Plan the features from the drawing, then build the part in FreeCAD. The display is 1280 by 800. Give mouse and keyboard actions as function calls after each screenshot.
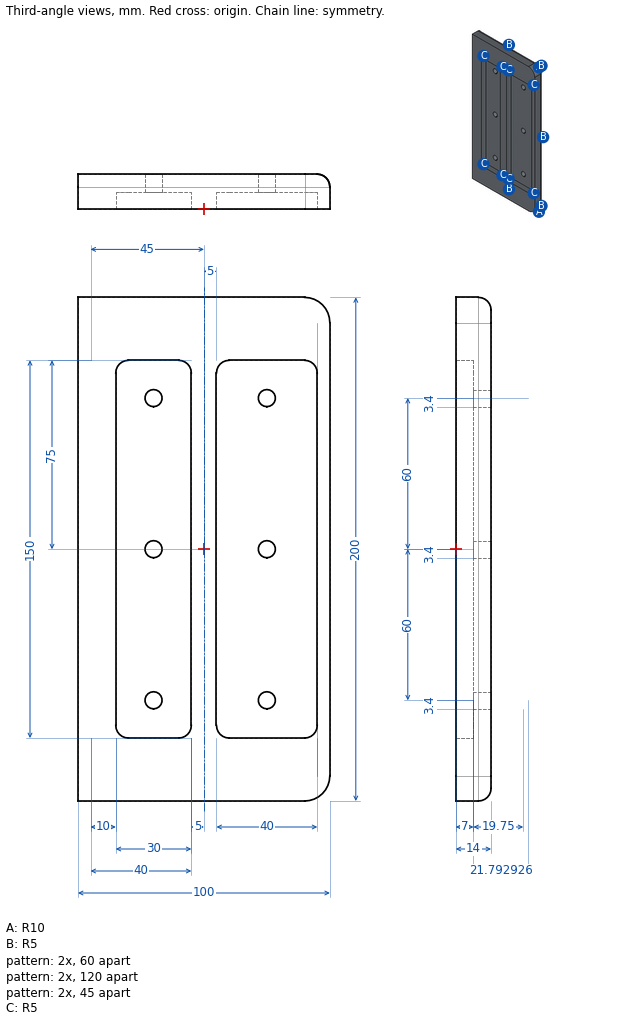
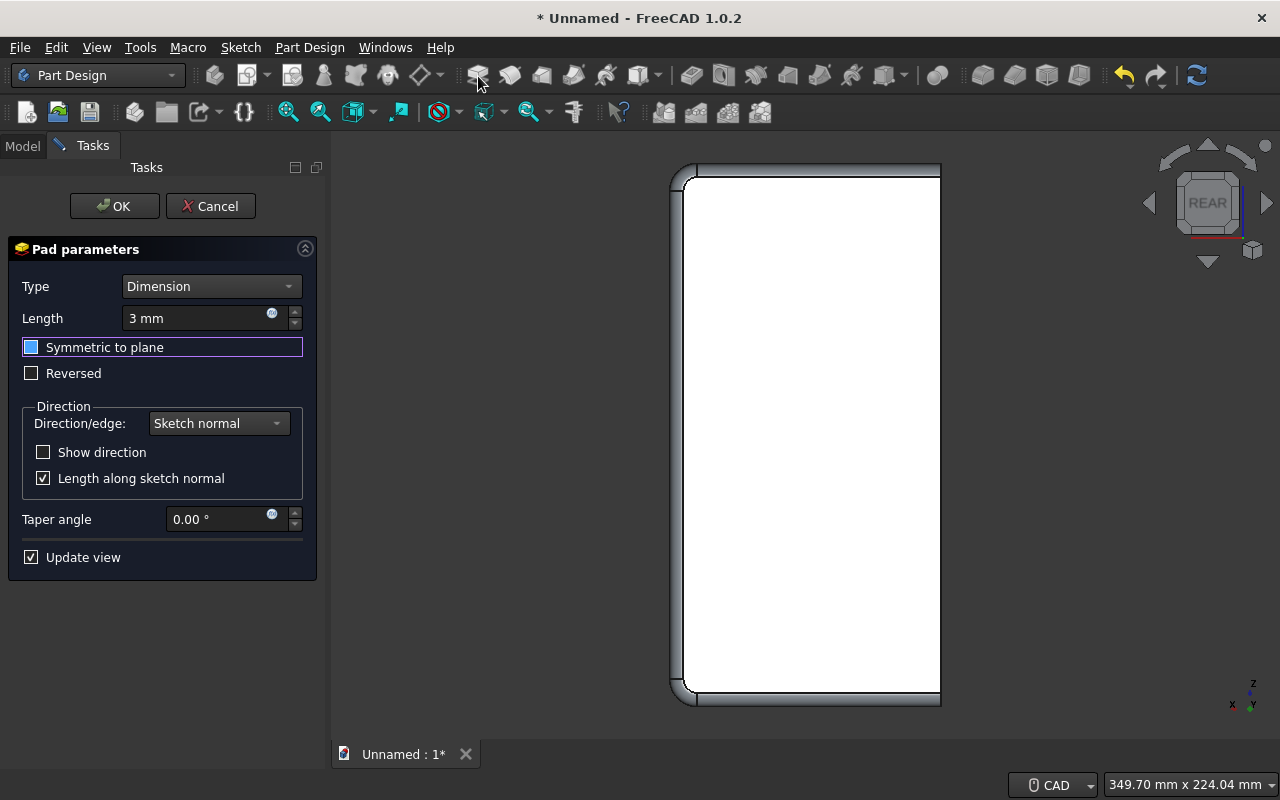
click(115, 206)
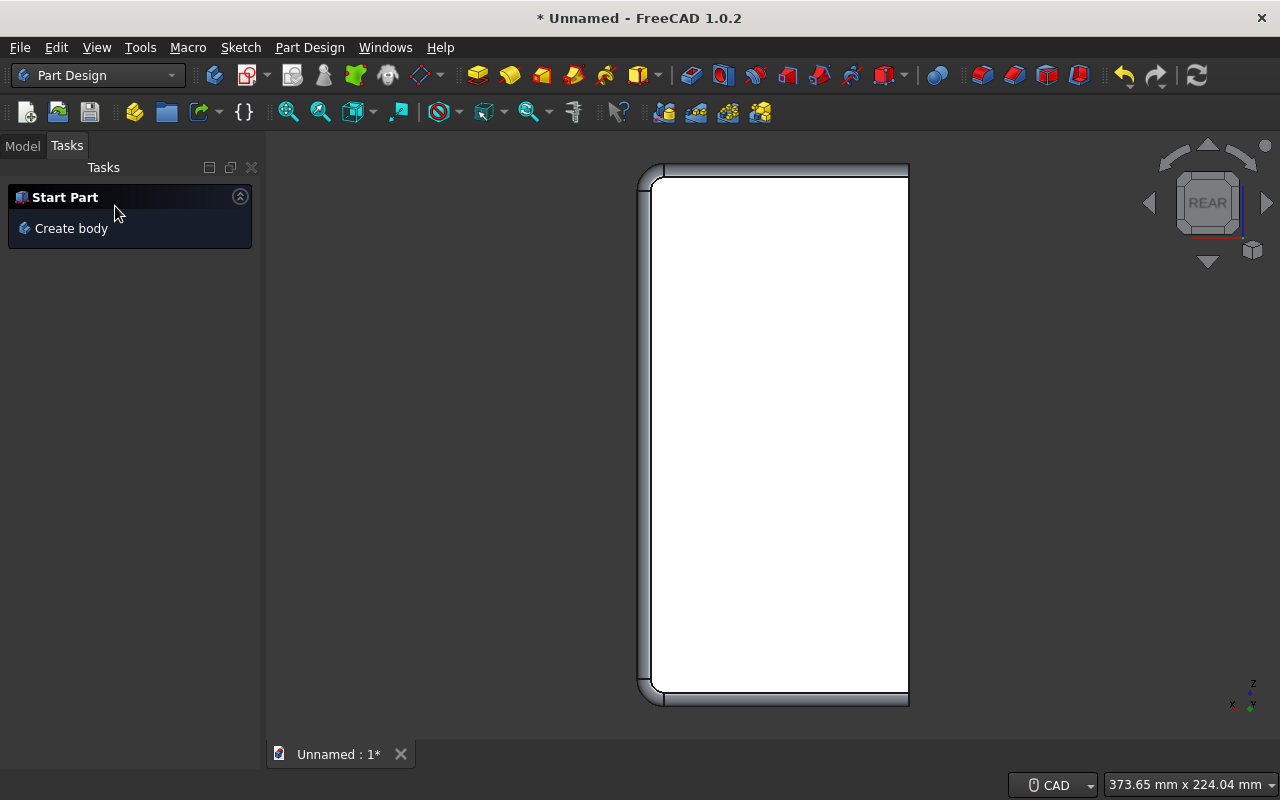
key(0)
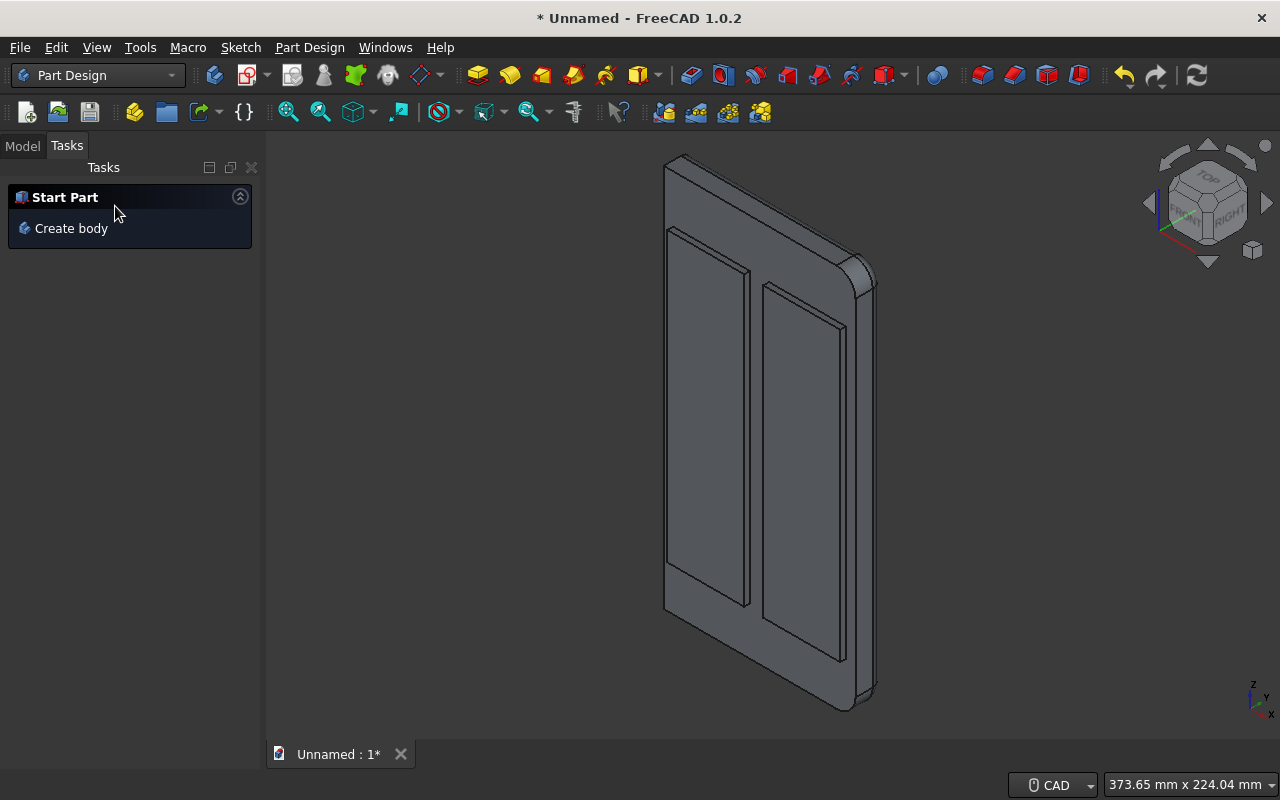
click(802, 378)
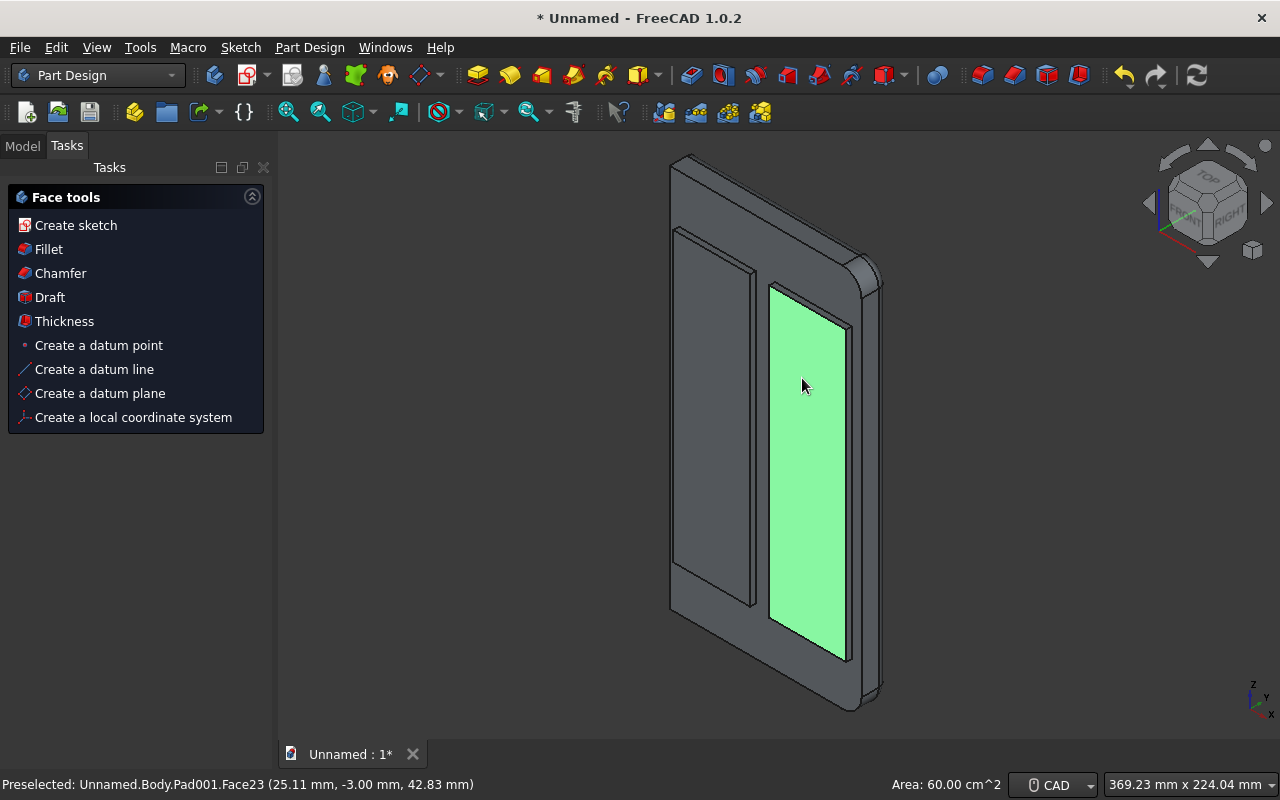
click(248, 76)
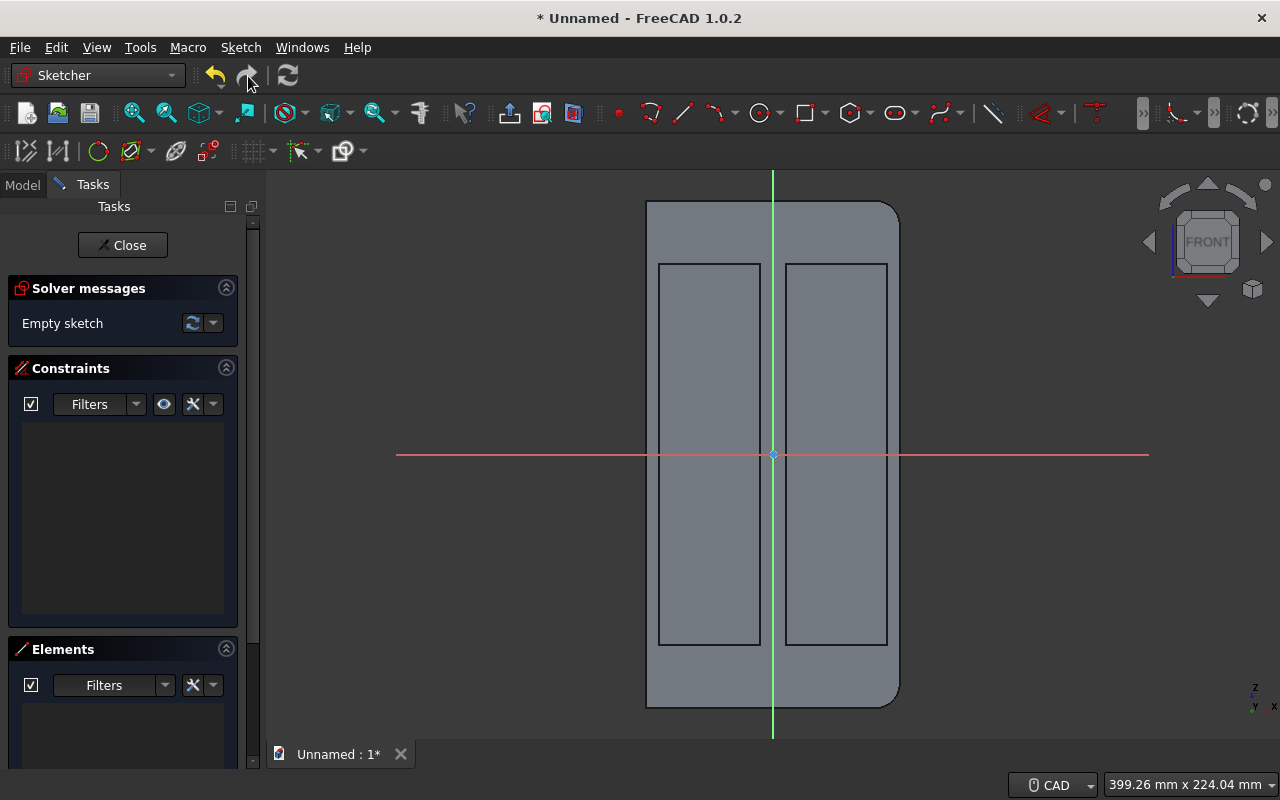
click(806, 114)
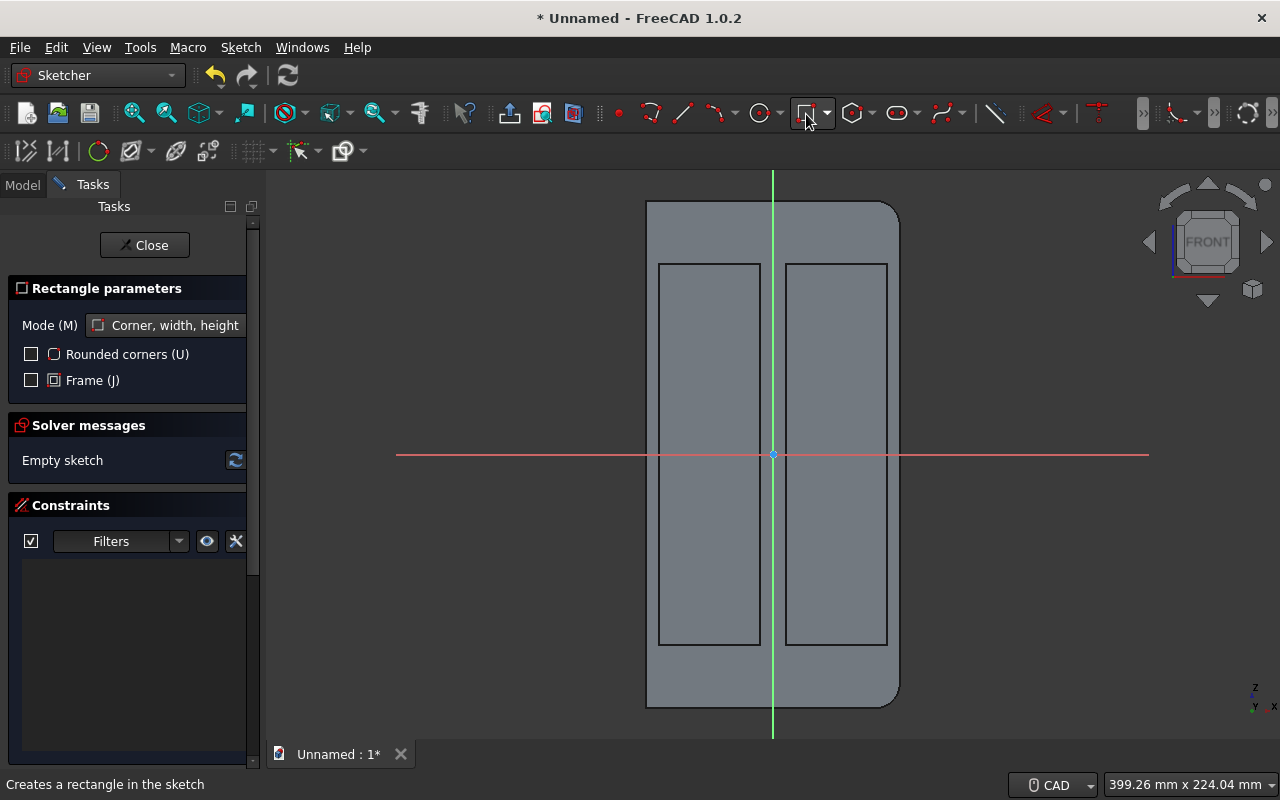
click(659, 264)
move(684, 645)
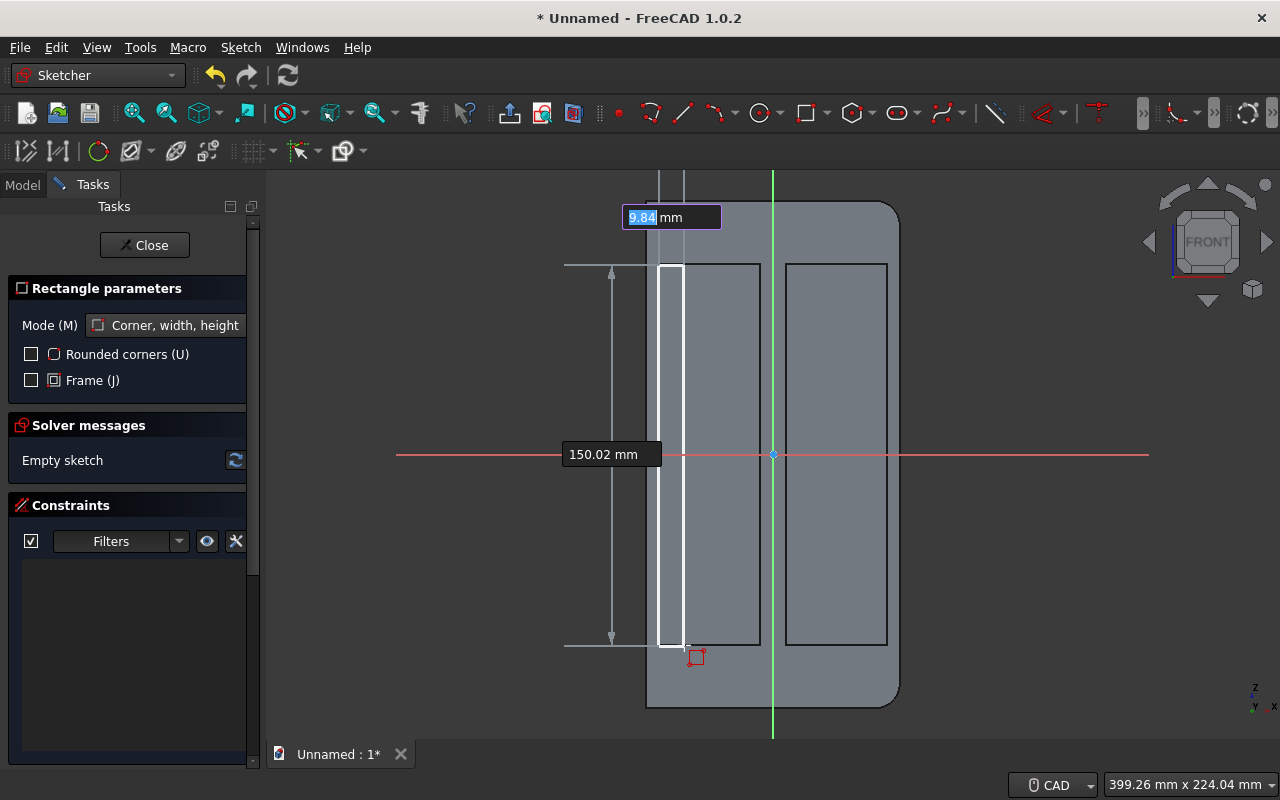
text(10)
key(Tab)
text(150)
key(Return)
key(Escape)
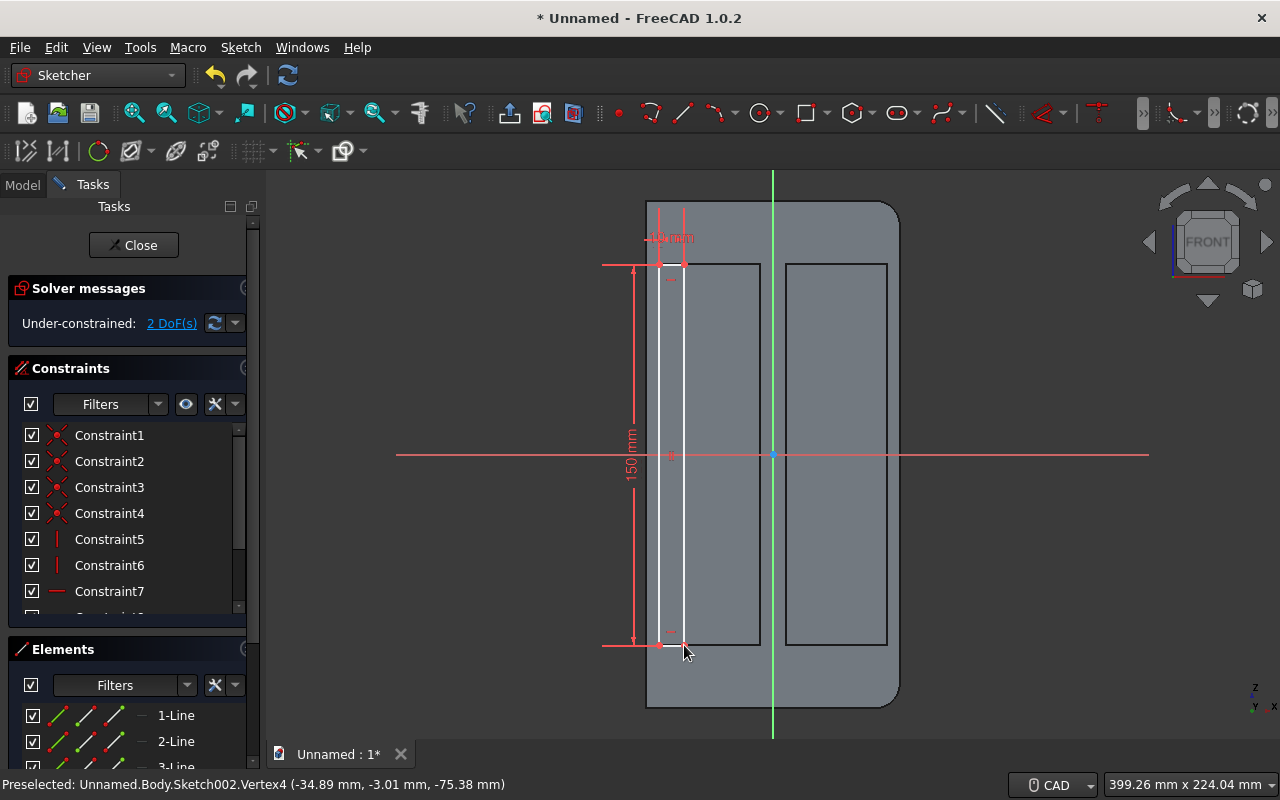
click(1042, 114)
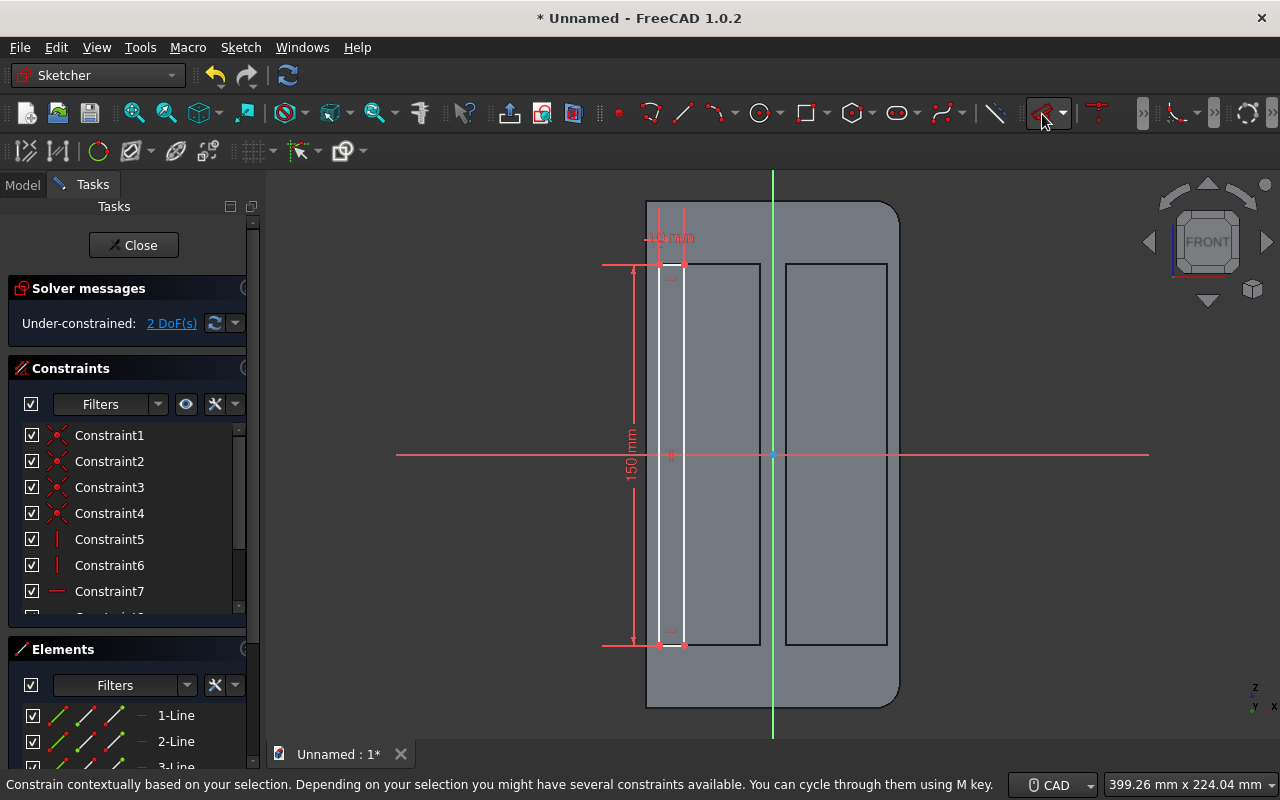
click(659, 265)
click(716, 231)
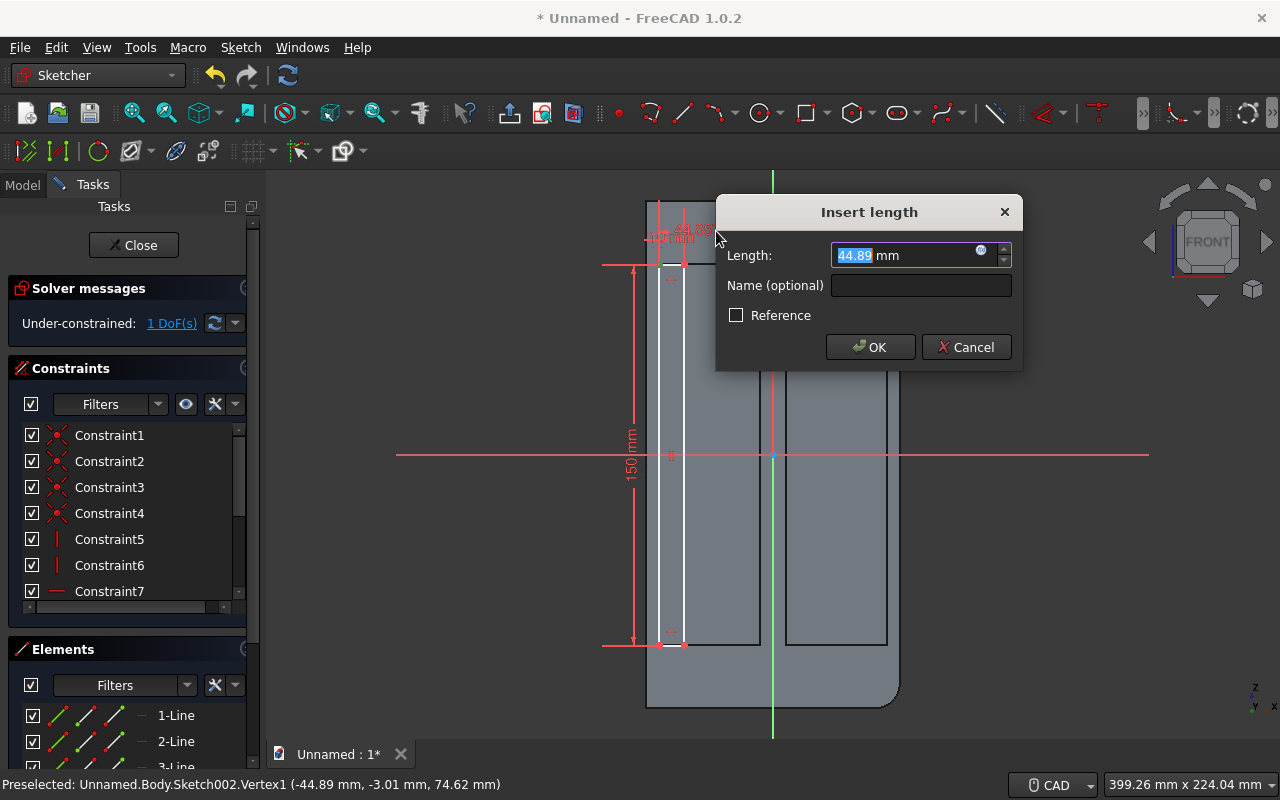
text(45)
key(Return)